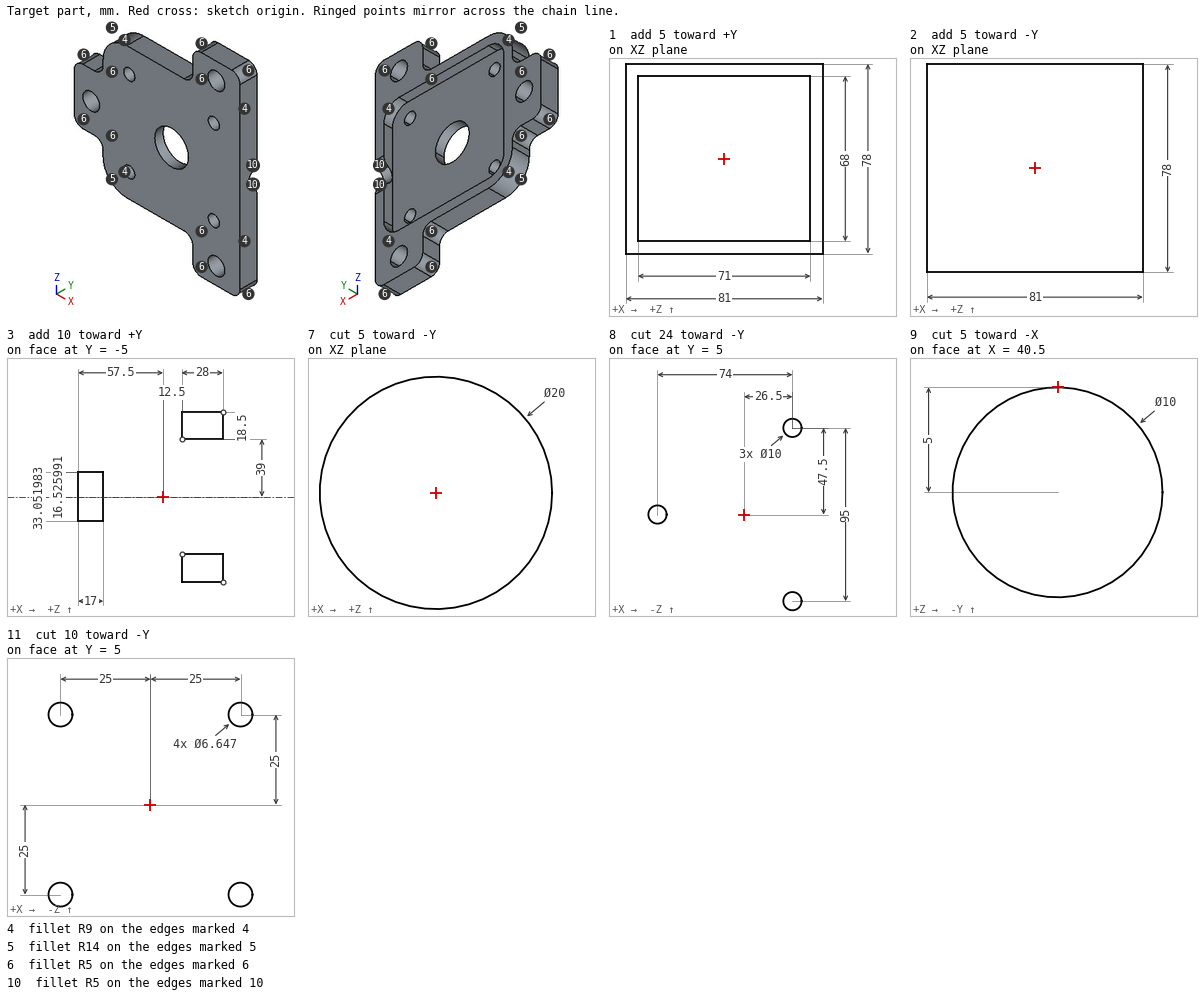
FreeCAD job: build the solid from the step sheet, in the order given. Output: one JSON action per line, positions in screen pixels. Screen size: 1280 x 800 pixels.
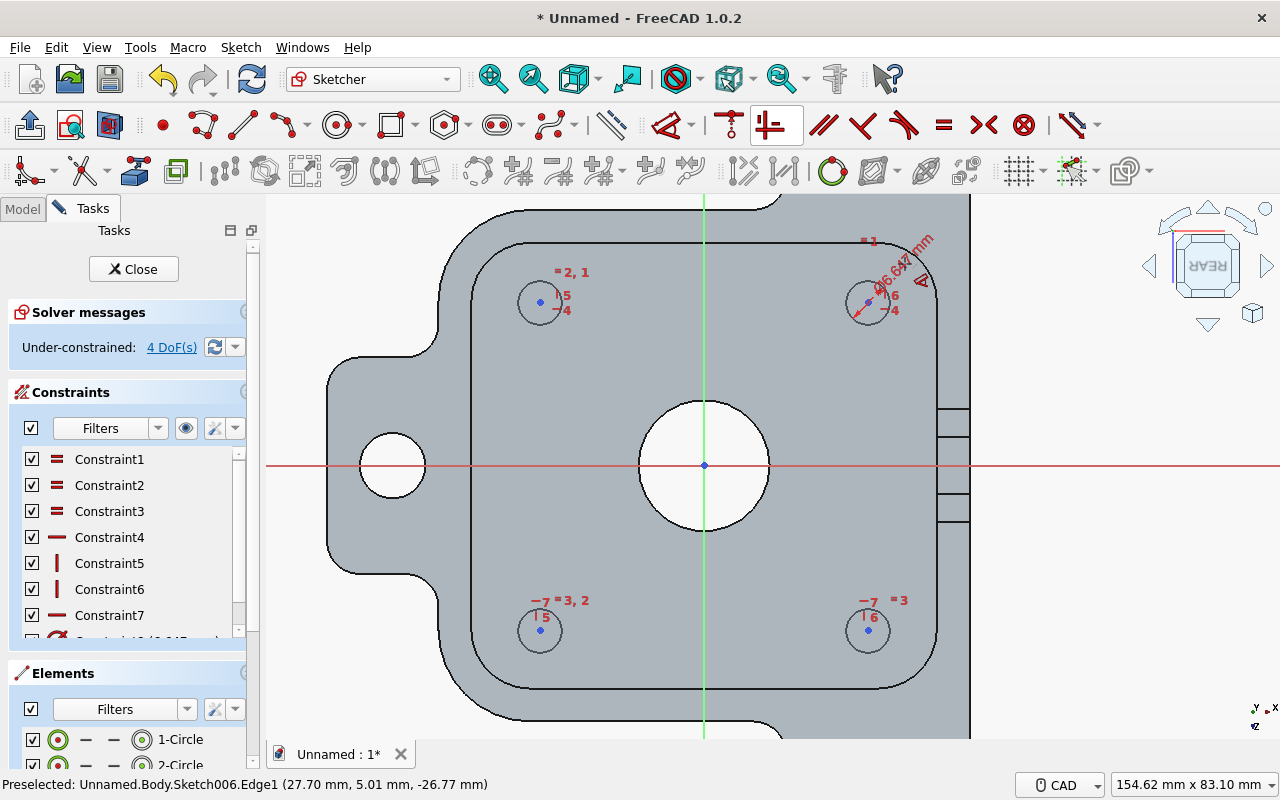
{"action": "left_click", "coordinate": [868, 303]}
{"action": "left_click", "coordinate": [786, 269]}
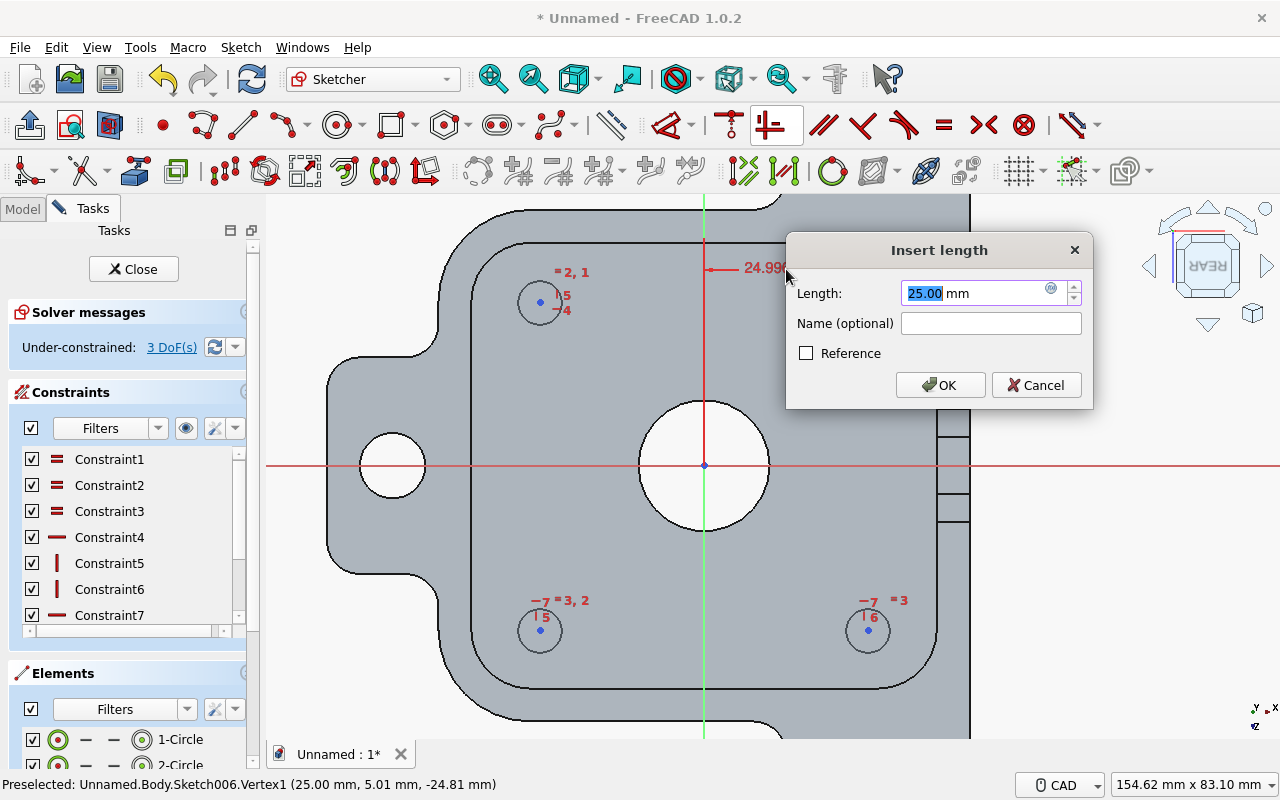
{"action": "type", "text": "25"}
{"action": "key", "text": "Return"}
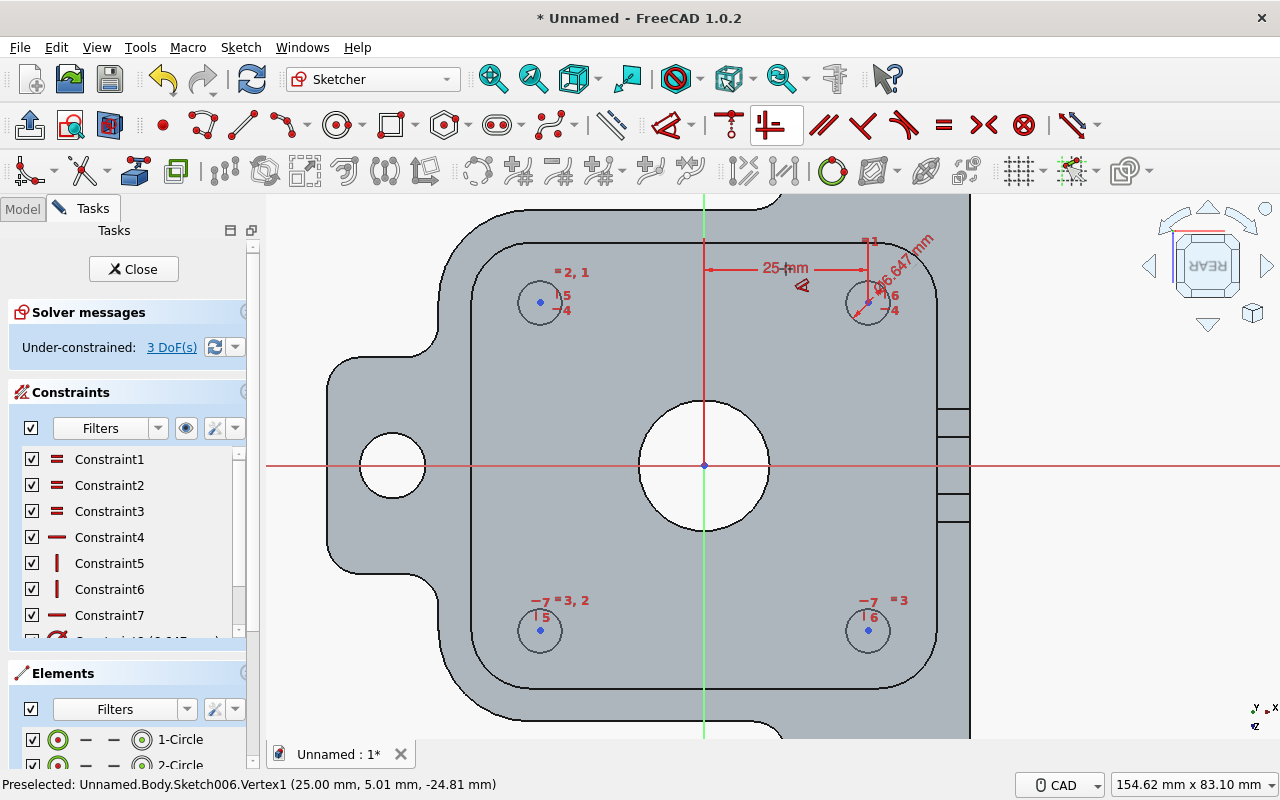
{"action": "left_click", "coordinate": [868, 303]}
{"action": "left_click", "coordinate": [902, 384]}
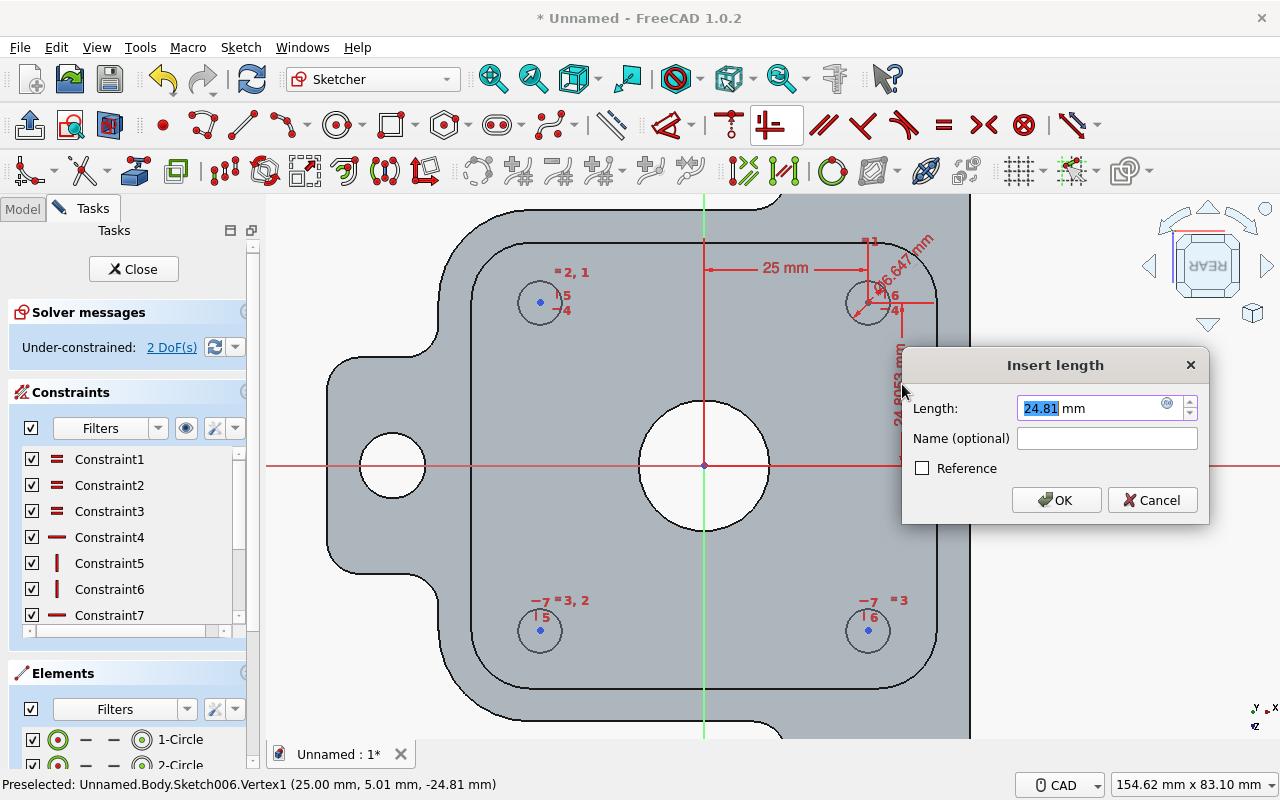
{"action": "type", "text": "25"}
{"action": "key", "text": "Return"}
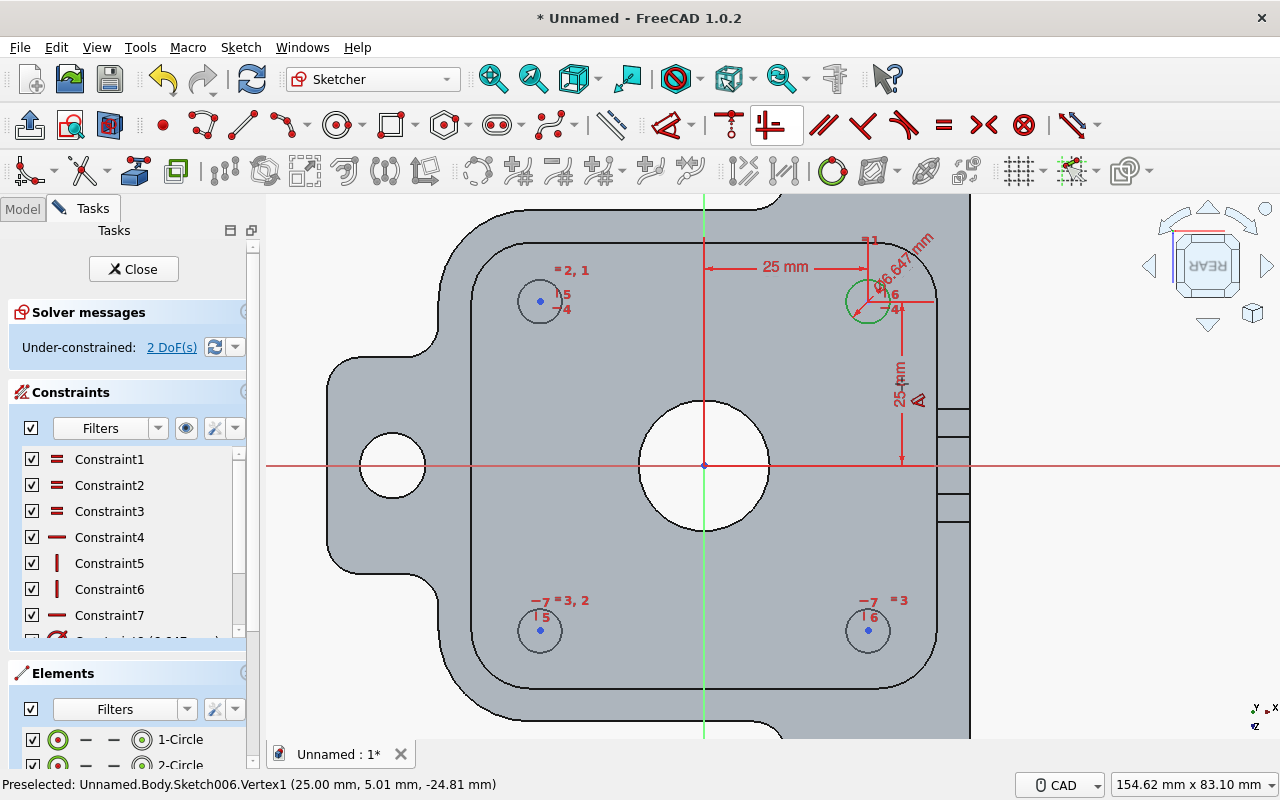
{"action": "left_click", "coordinate": [540, 302]}
{"action": "left_click", "coordinate": [622, 268]}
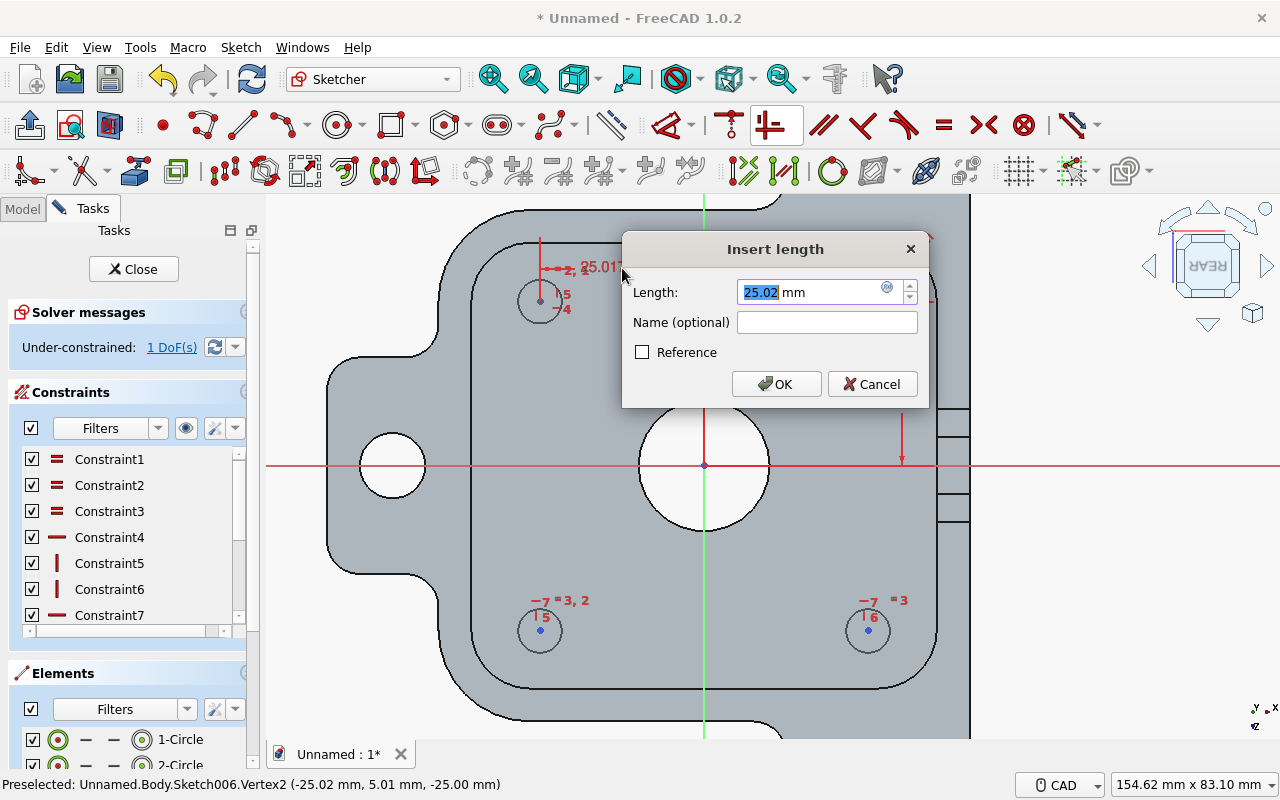
{"action": "type", "text": "25"}
{"action": "key", "text": "Return"}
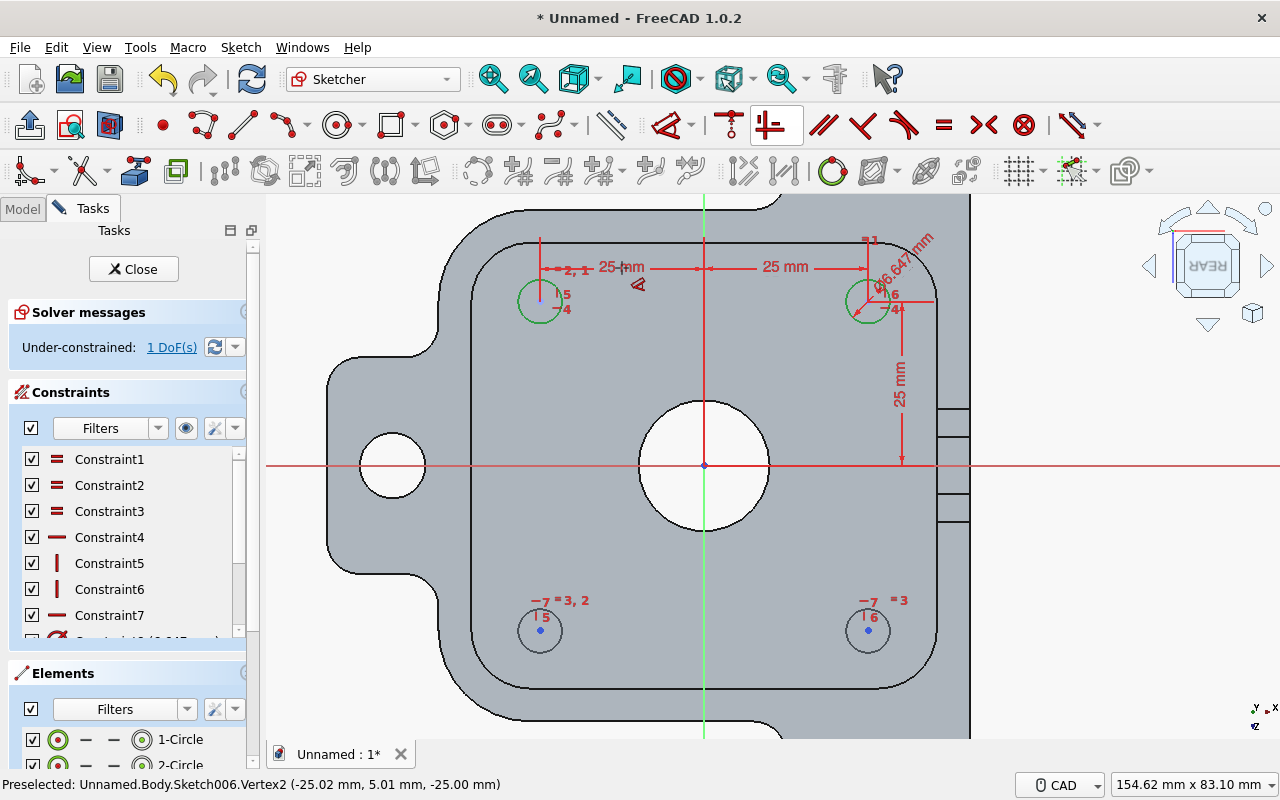
{"action": "left_click", "coordinate": [540, 631]}
{"action": "left_click", "coordinate": [506, 548]}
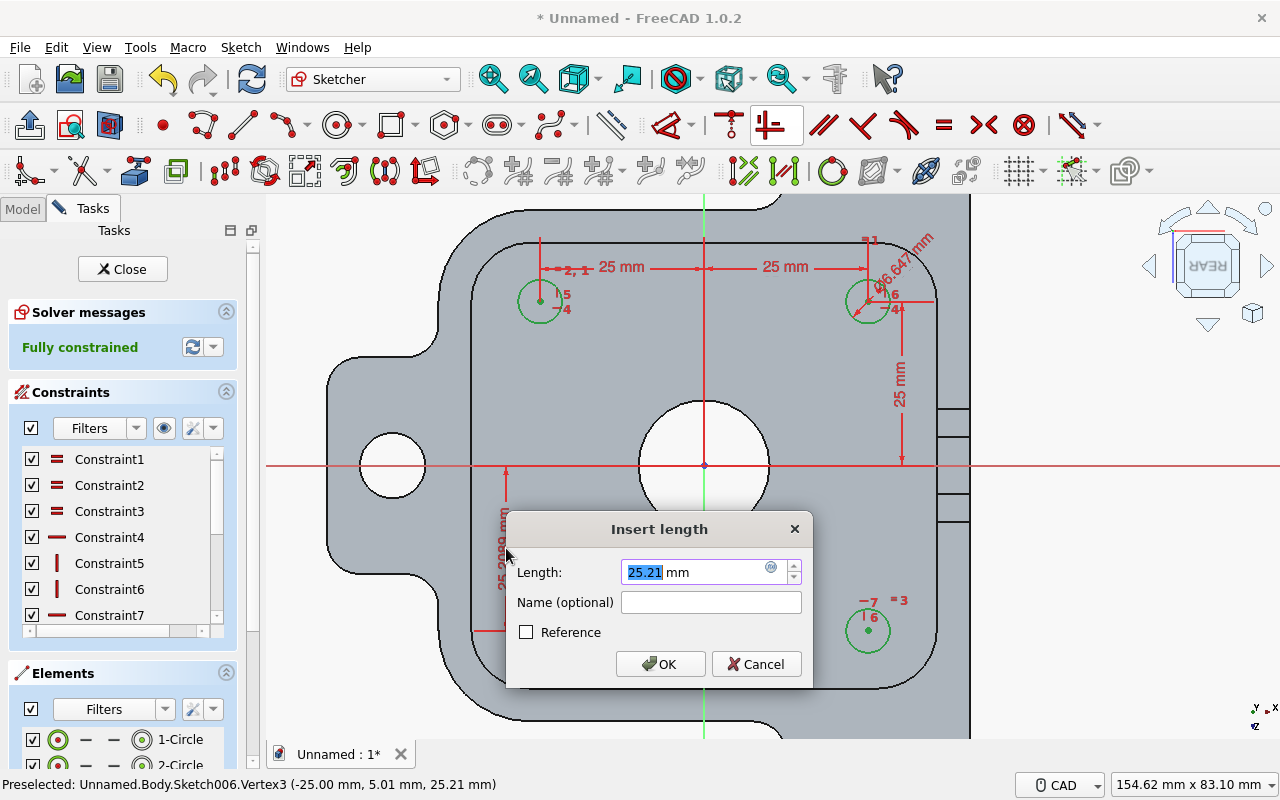
{"action": "type", "text": "25"}
{"action": "key", "text": "Return"}
{"action": "key", "text": "Escape"}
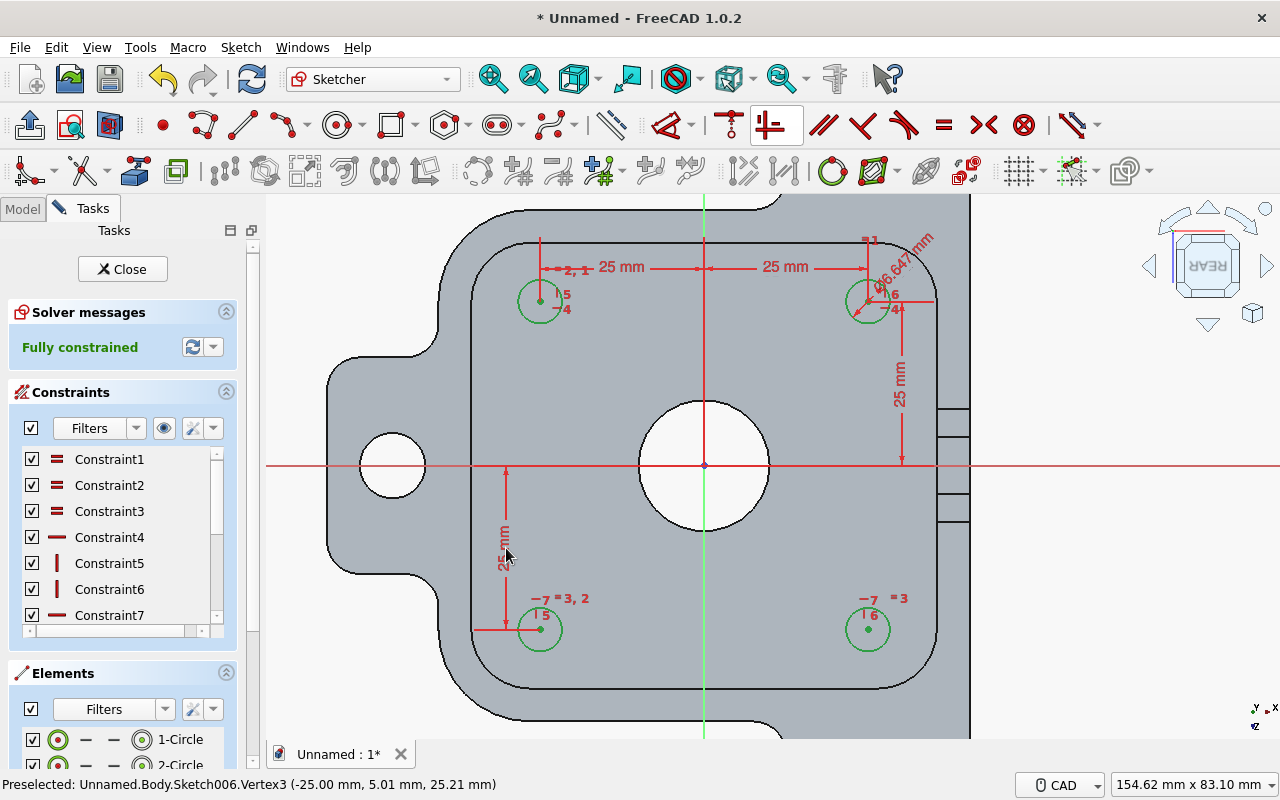
{"action": "left_click", "coordinate": [123, 269]}